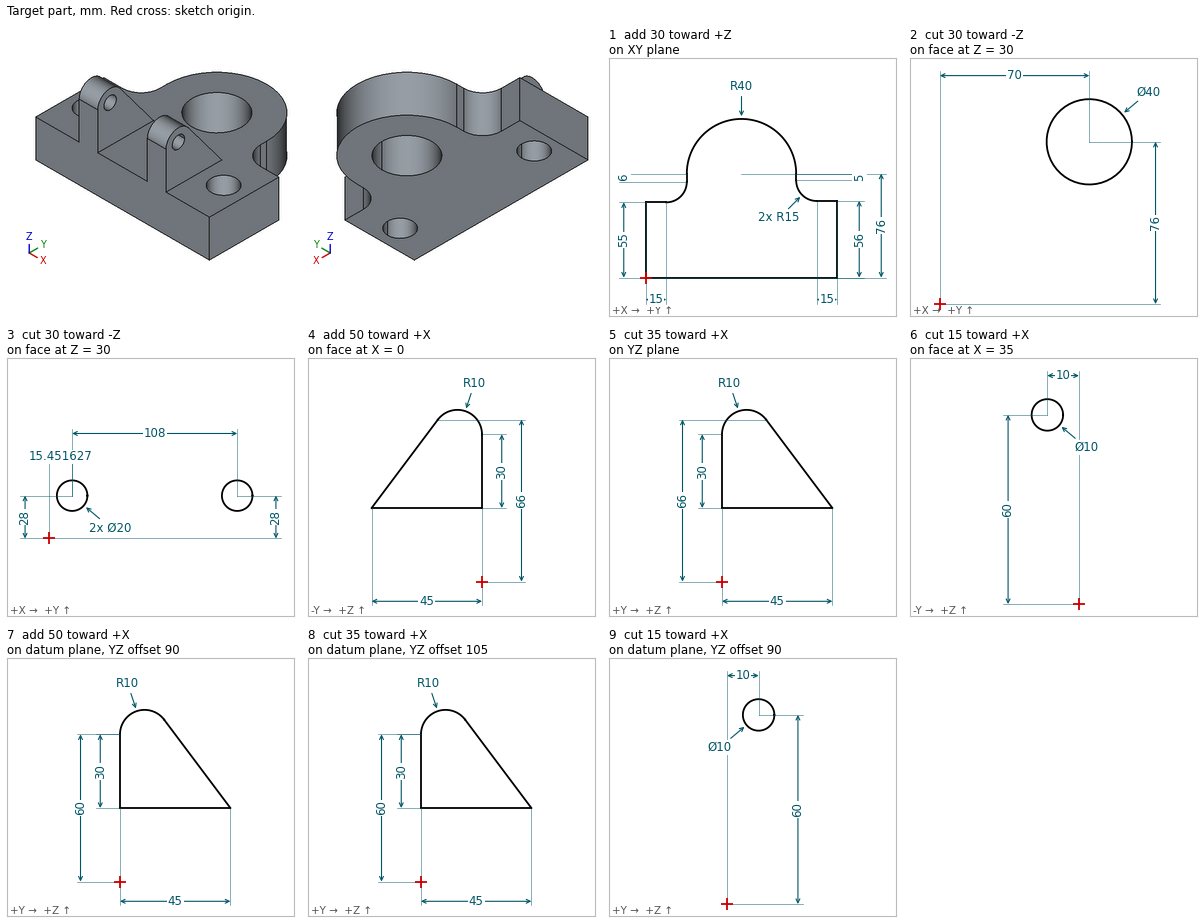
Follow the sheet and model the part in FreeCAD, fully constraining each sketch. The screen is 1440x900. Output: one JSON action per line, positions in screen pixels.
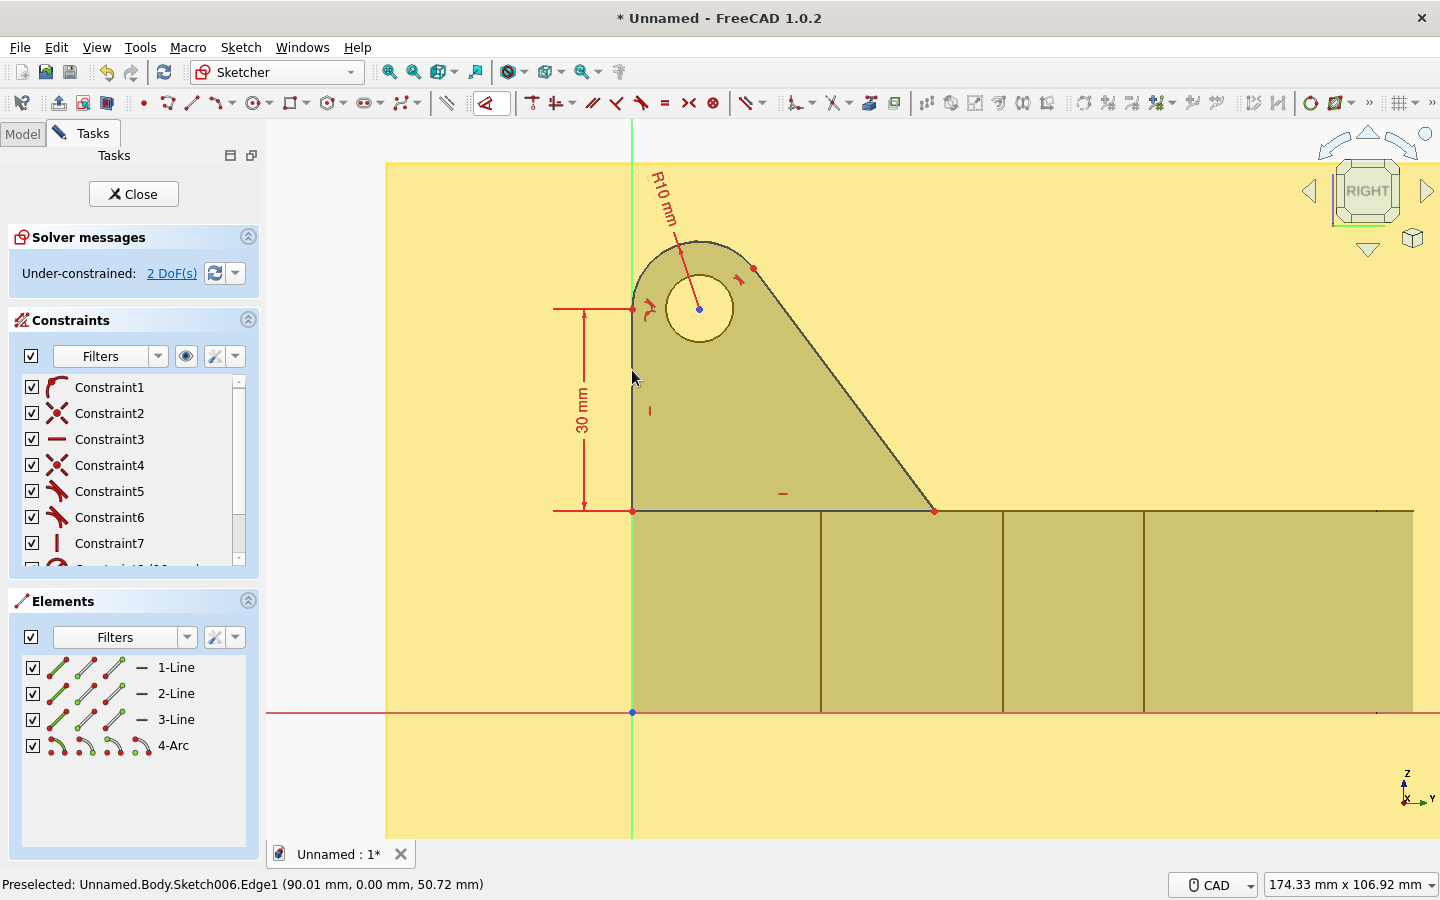
{"action": "left_click", "coordinate": [723, 511]}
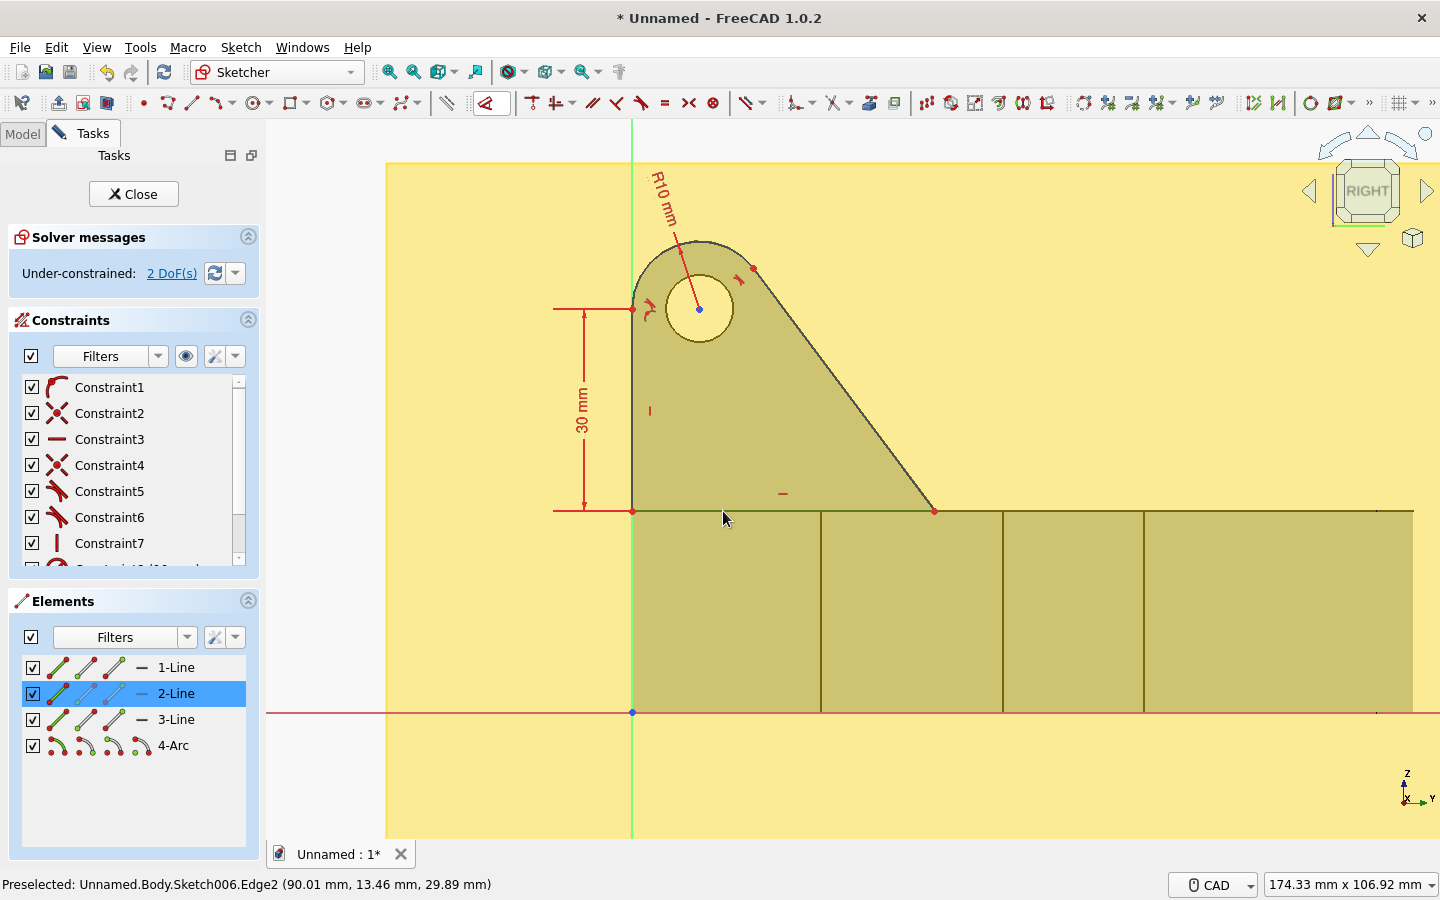
{"action": "left_click", "coordinate": [504, 104]}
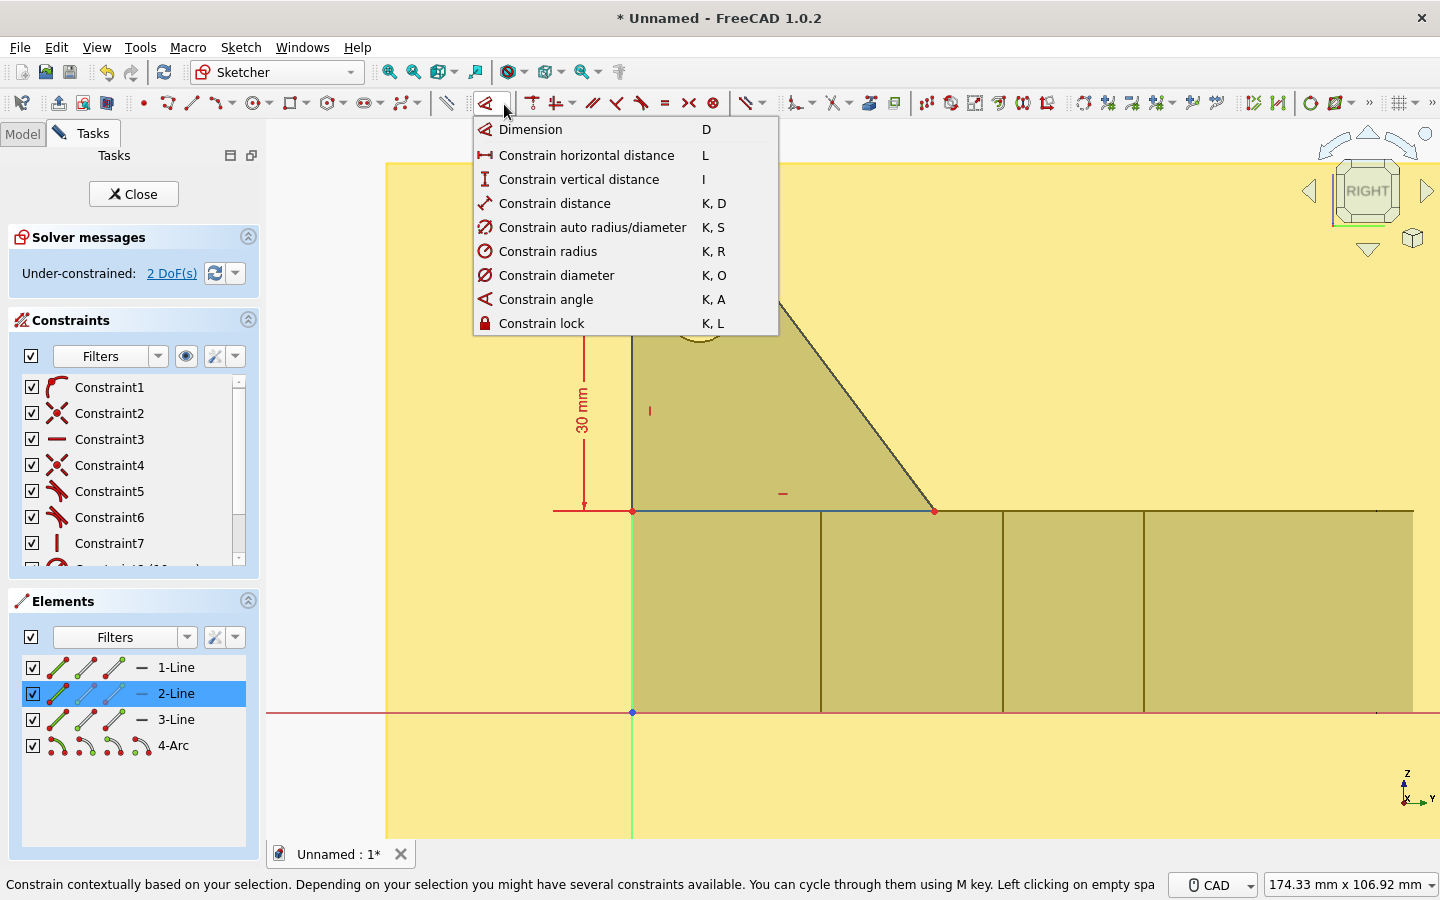
{"action": "left_click", "coordinate": [626, 155]}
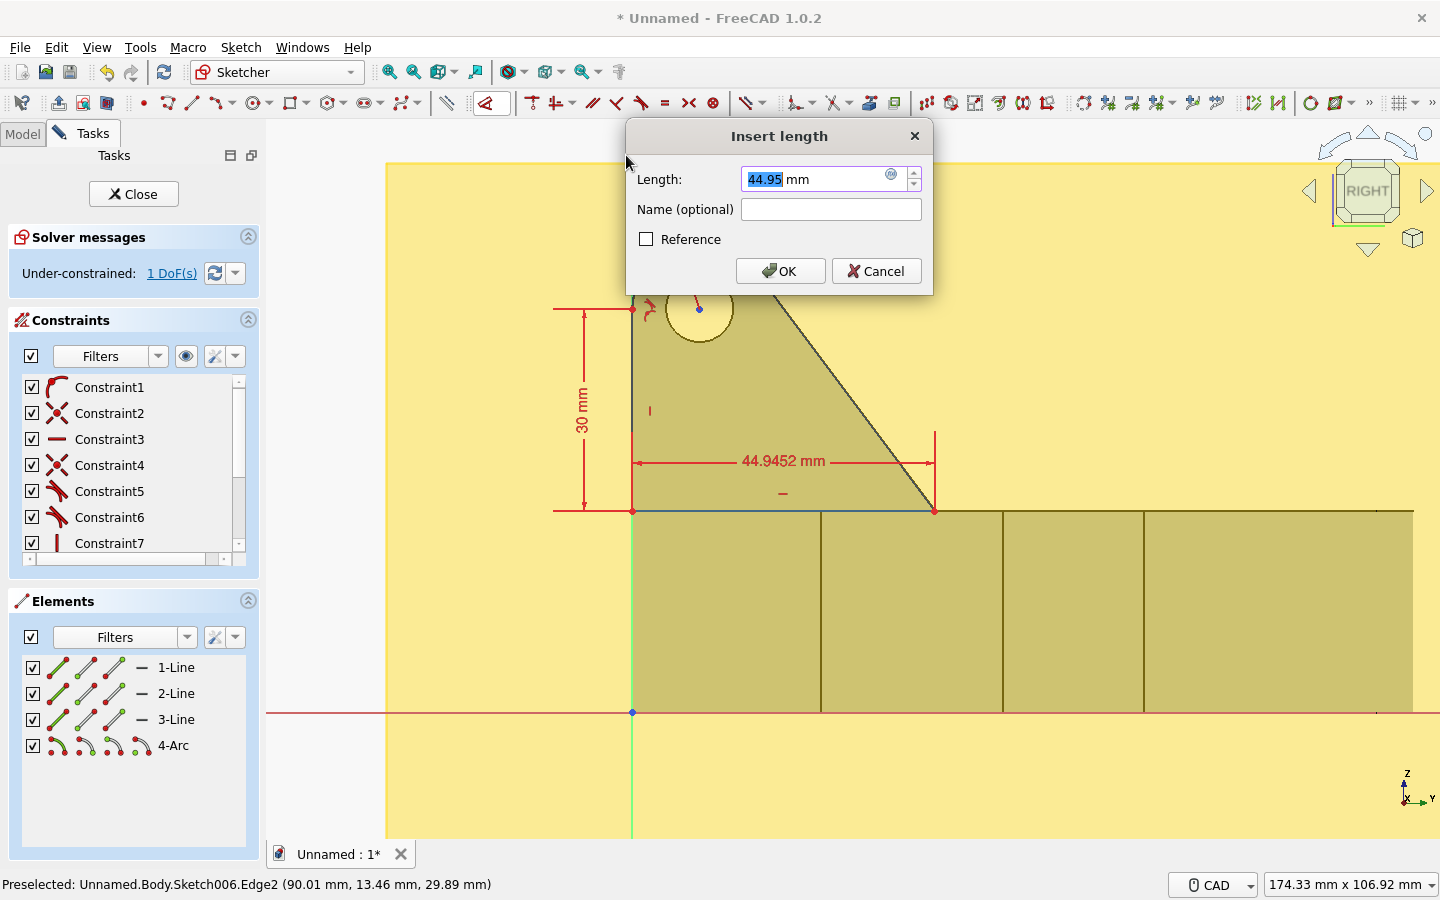
{"action": "type", "text": "45"}
{"action": "key", "text": "Return"}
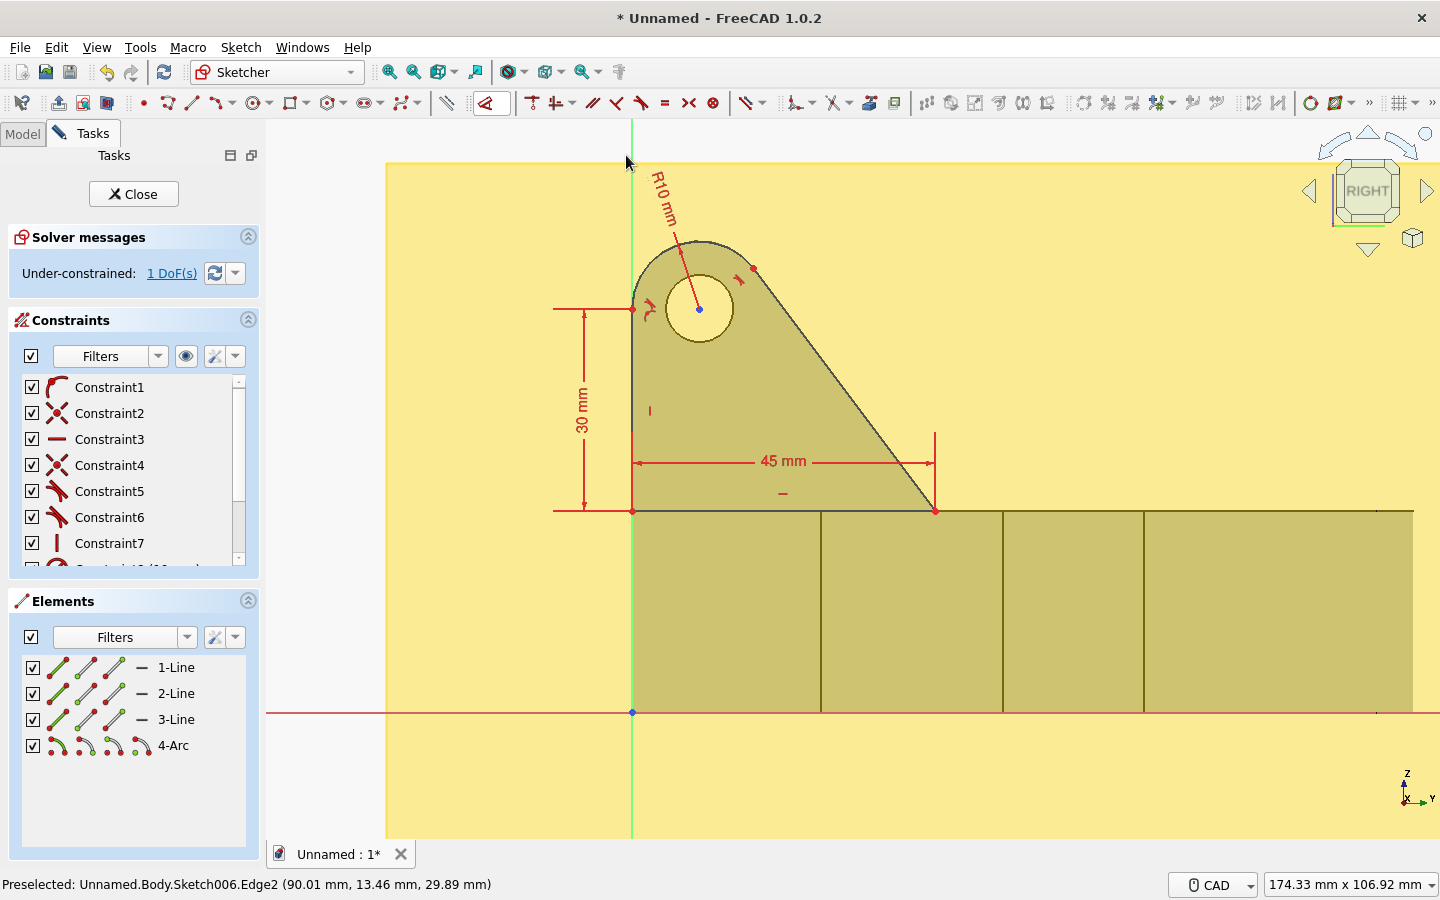
{"action": "left_click", "coordinate": [632, 309]}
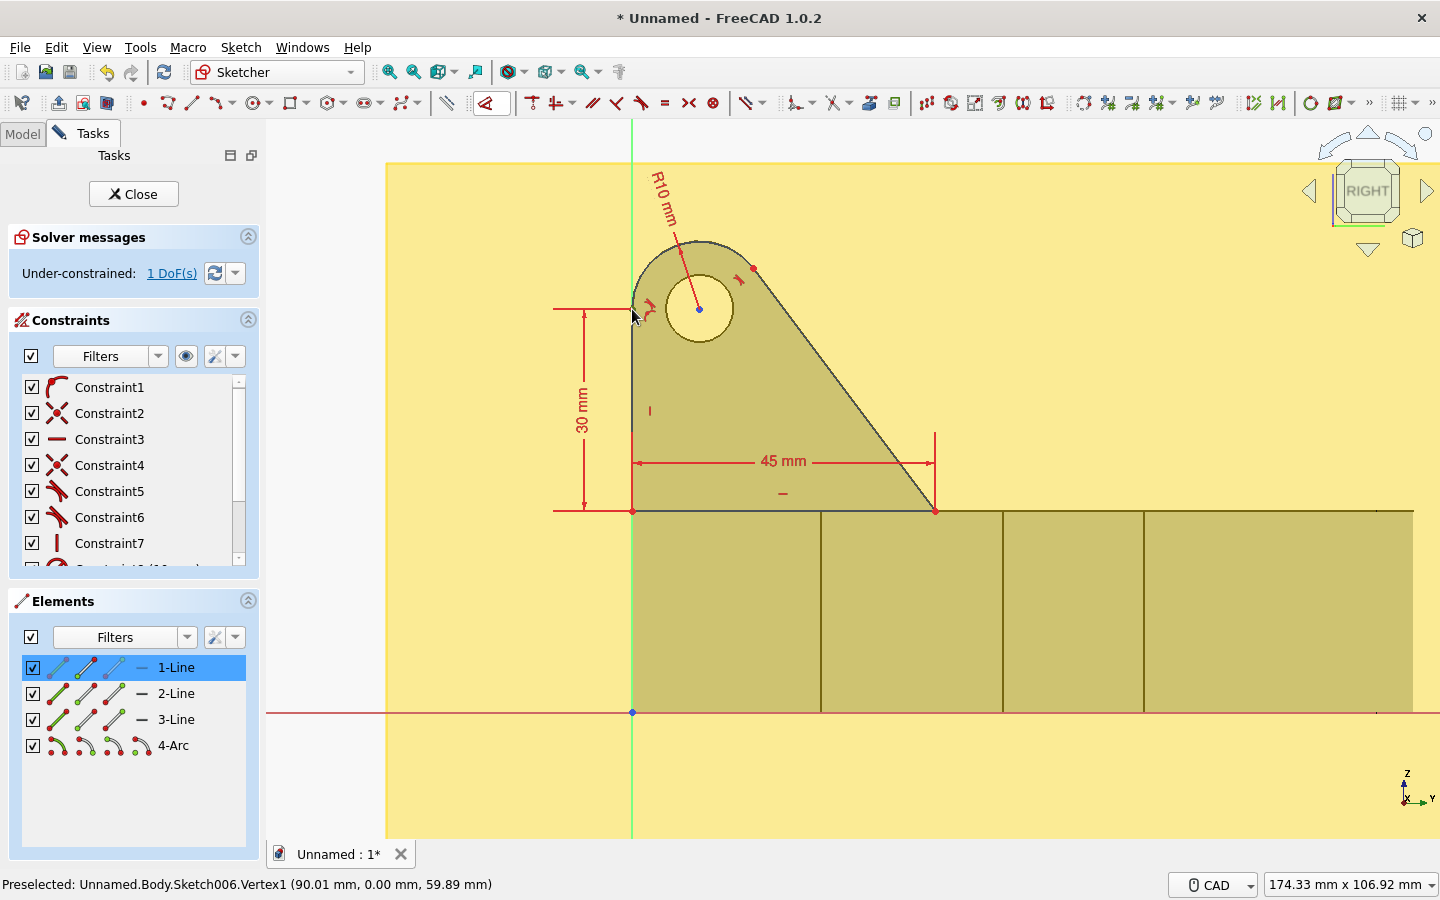
{"action": "key", "text": "i"}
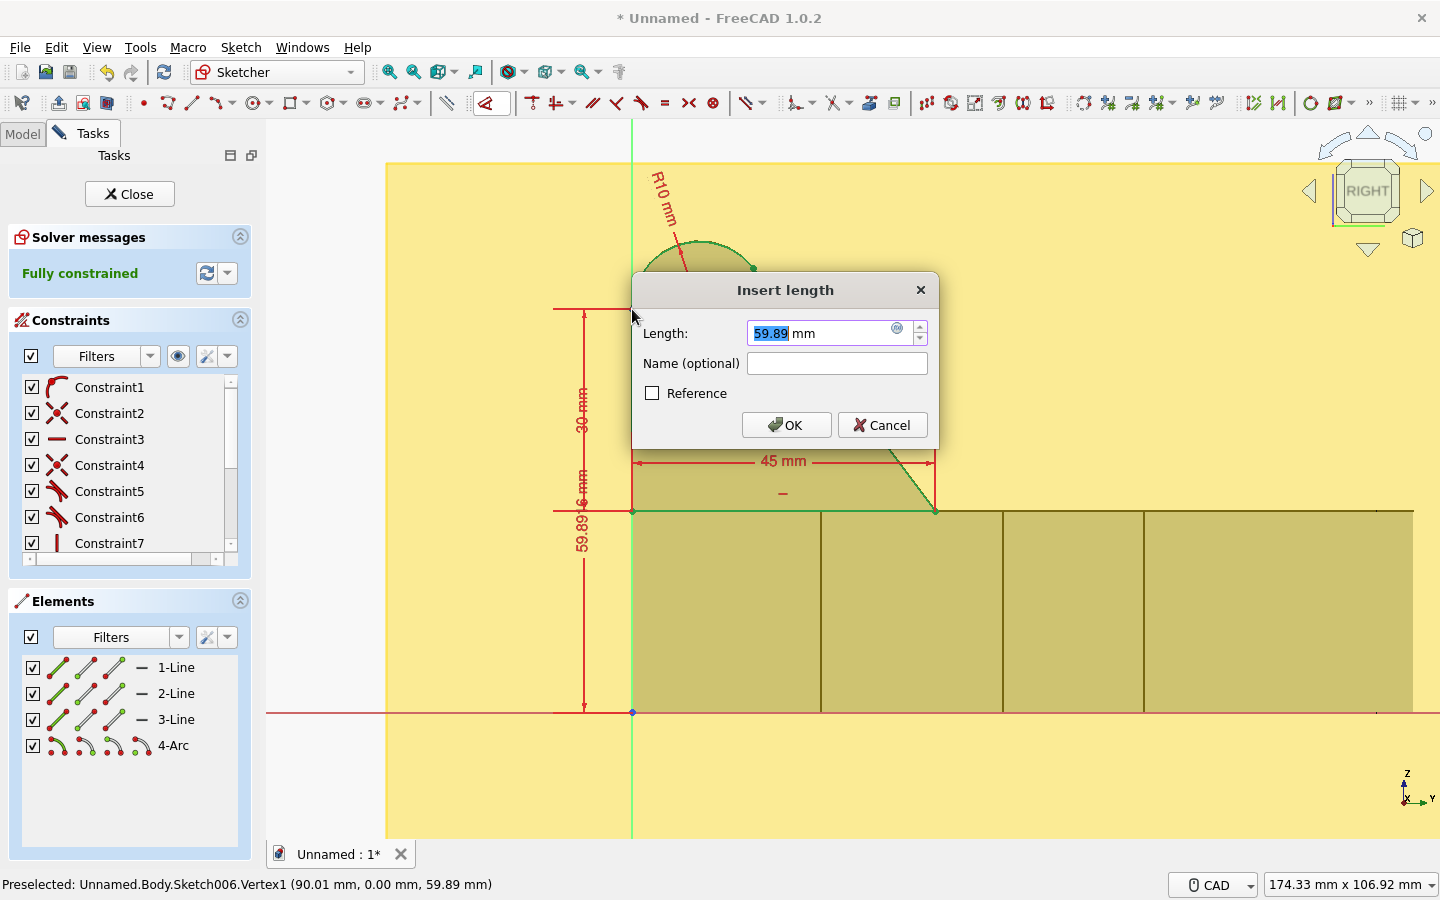
{"action": "type", "text": "60"}
{"action": "key", "text": "Return"}